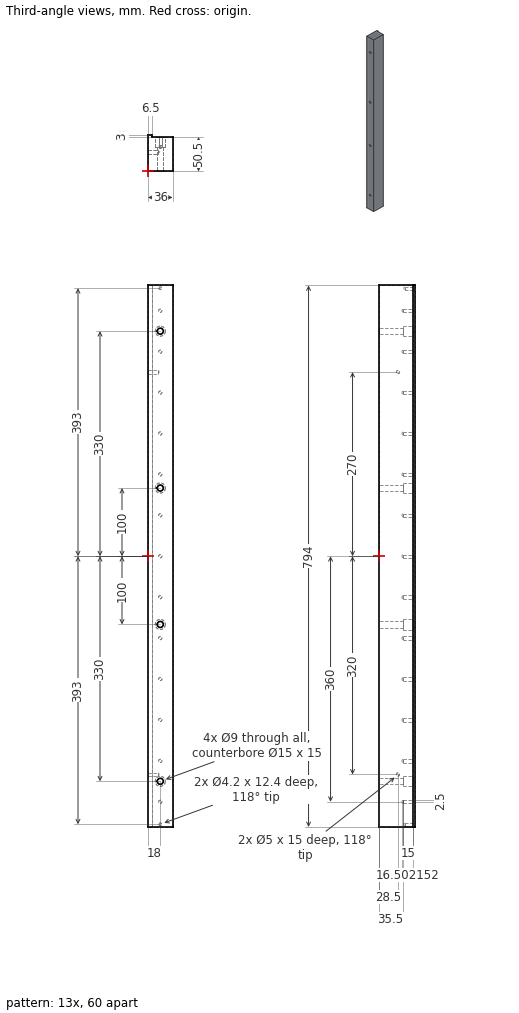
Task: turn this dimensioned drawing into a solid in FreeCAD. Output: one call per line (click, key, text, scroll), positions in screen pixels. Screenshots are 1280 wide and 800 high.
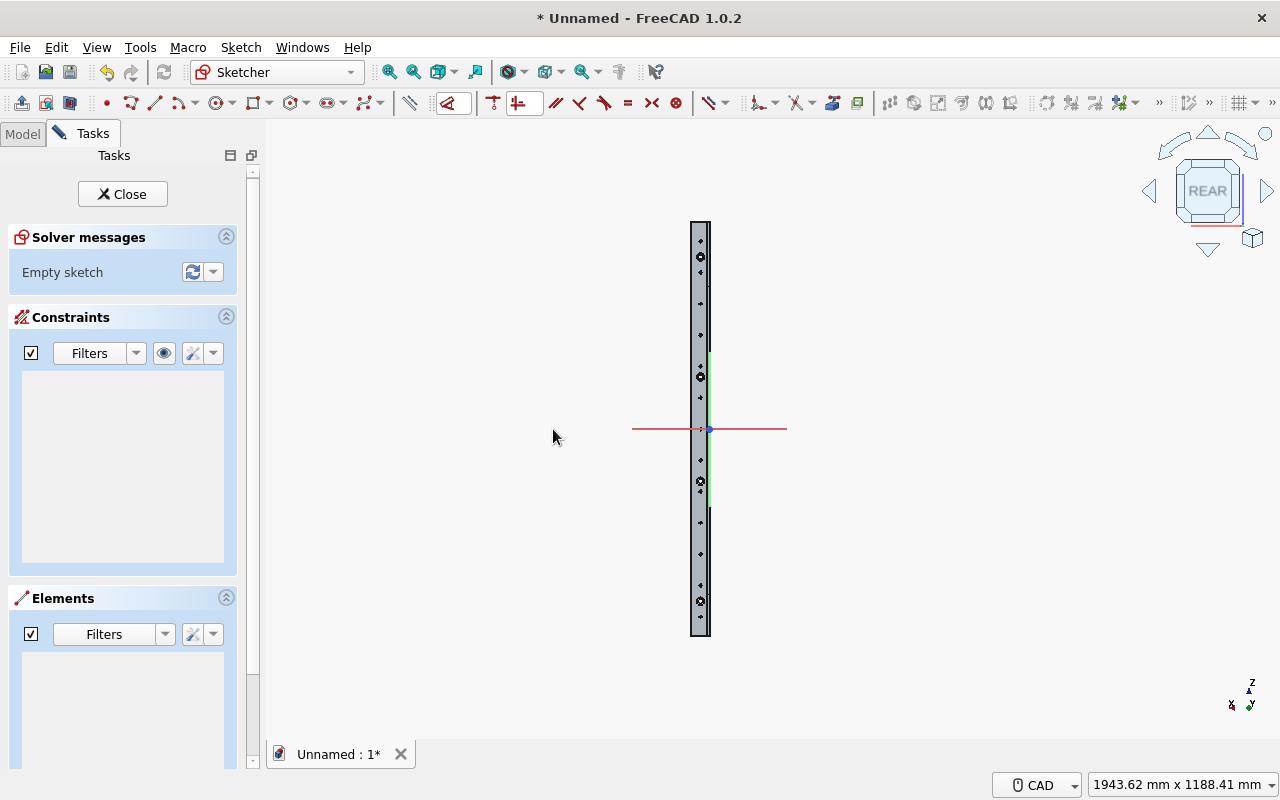
click(216, 104)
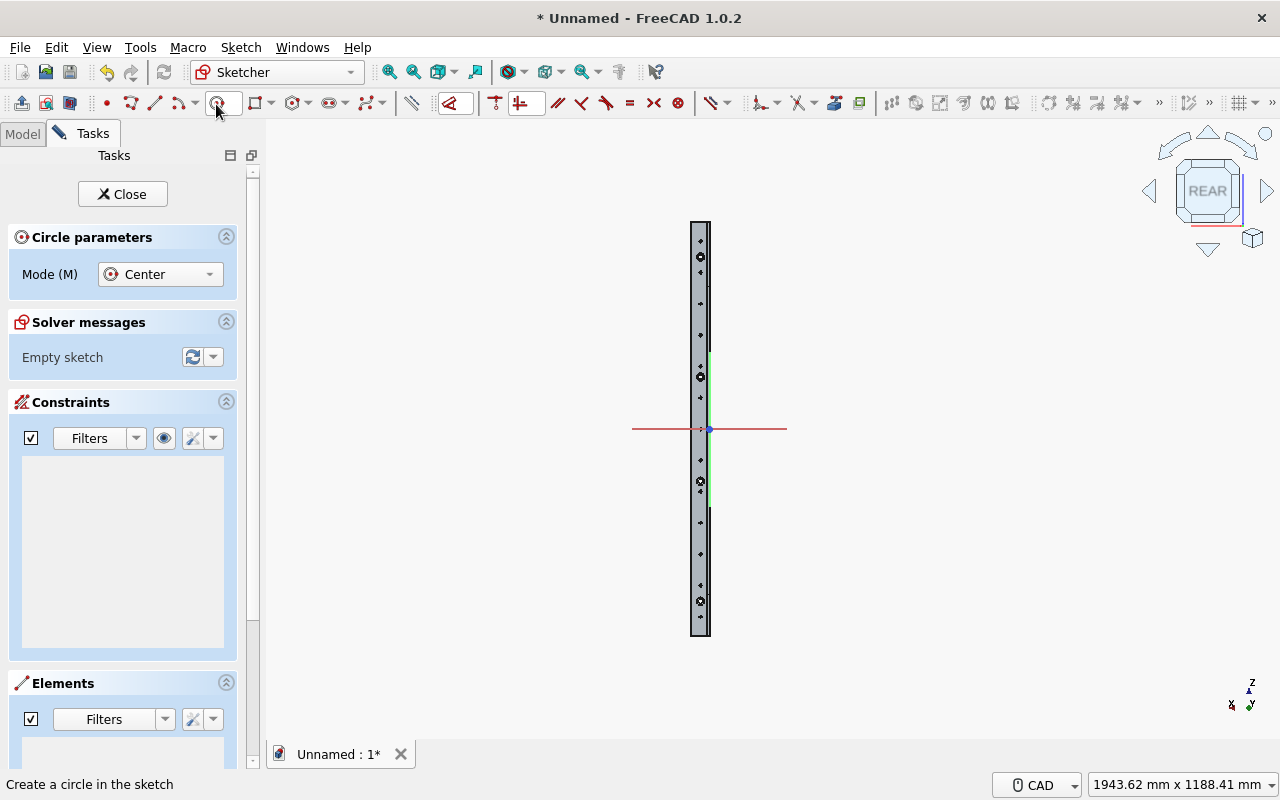
scroll(701, 634, up, 16)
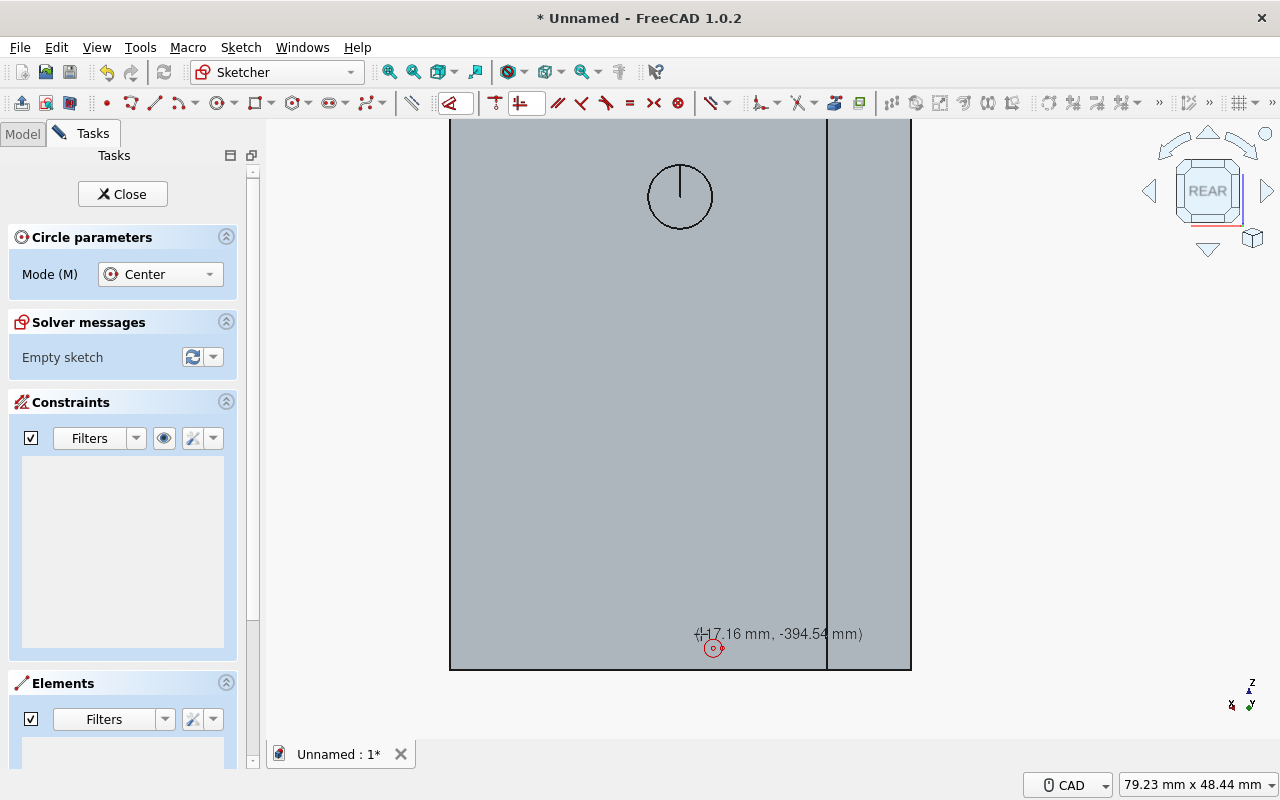
scroll(700, 683, down, 15)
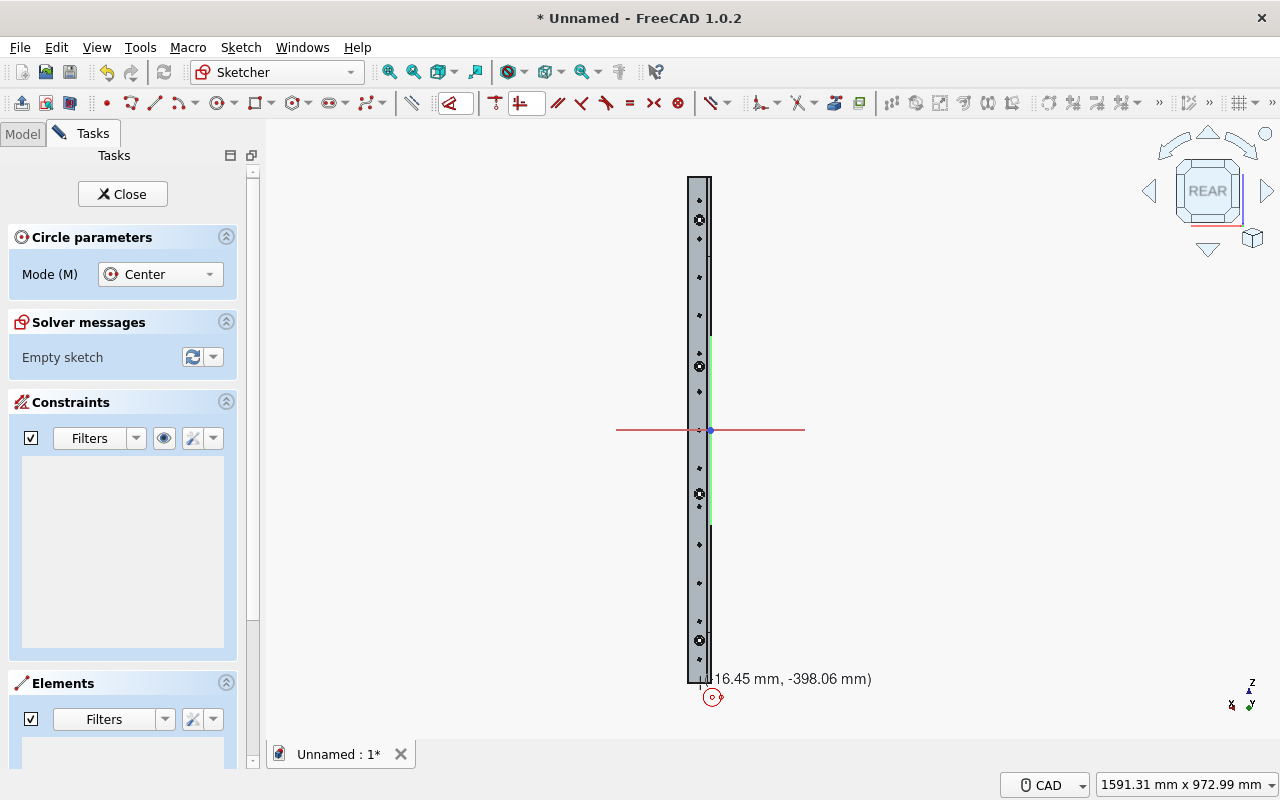
scroll(699, 681, up, 2)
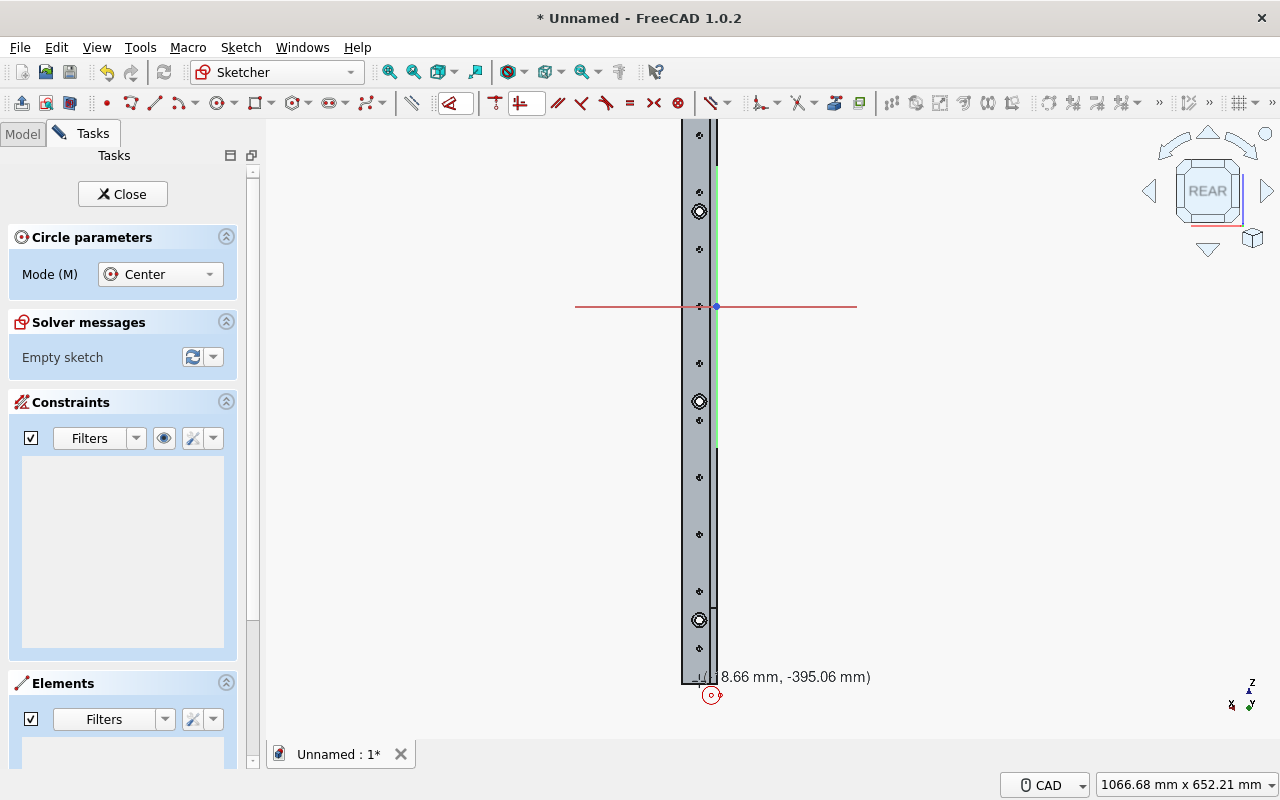
click(699, 680)
move(701, 679)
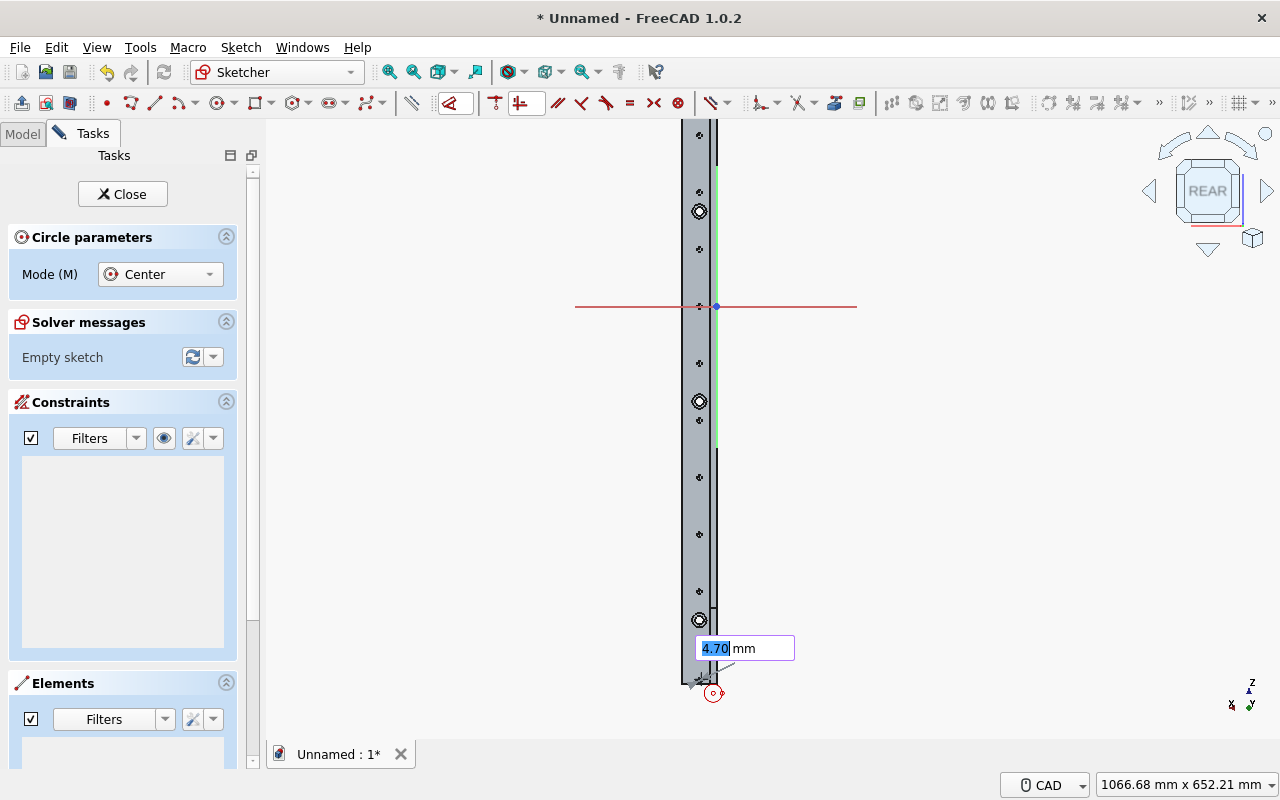
text(4.2)
key(Return)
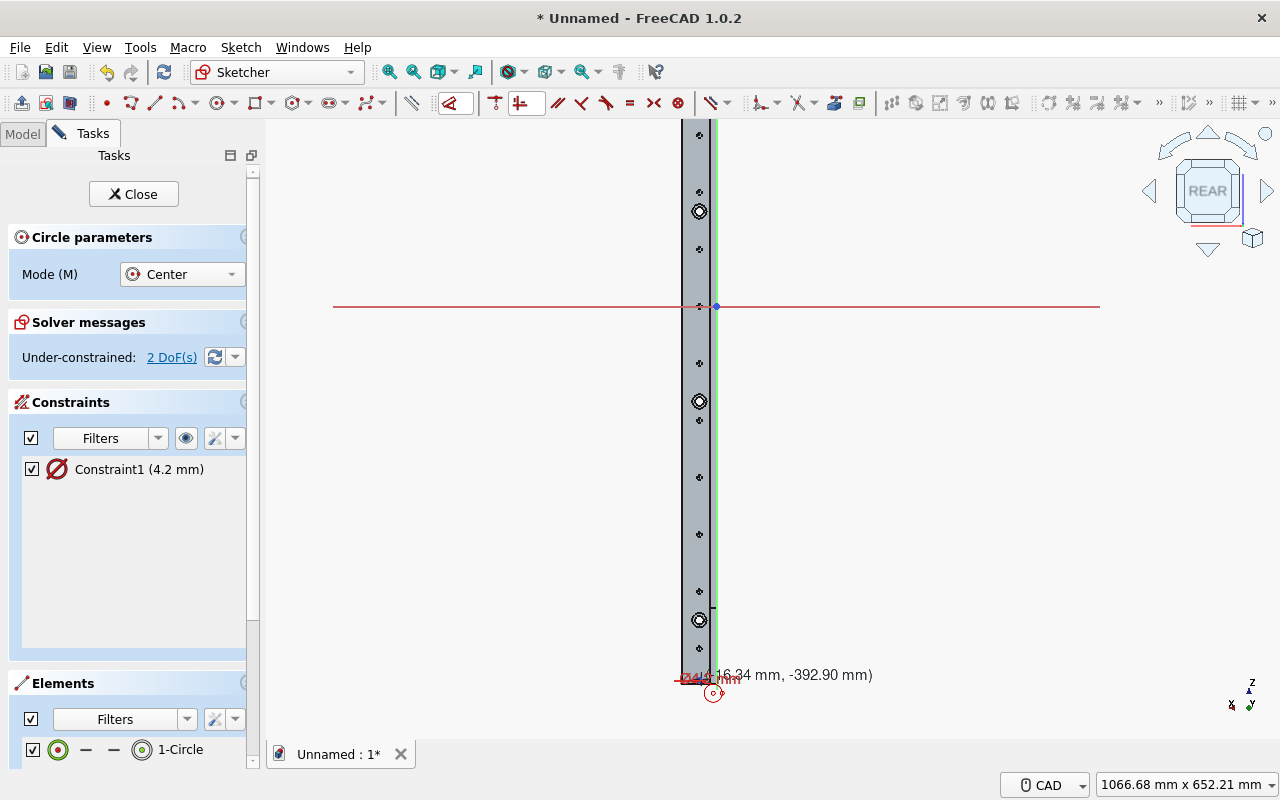
scroll(701, 578, down, 3)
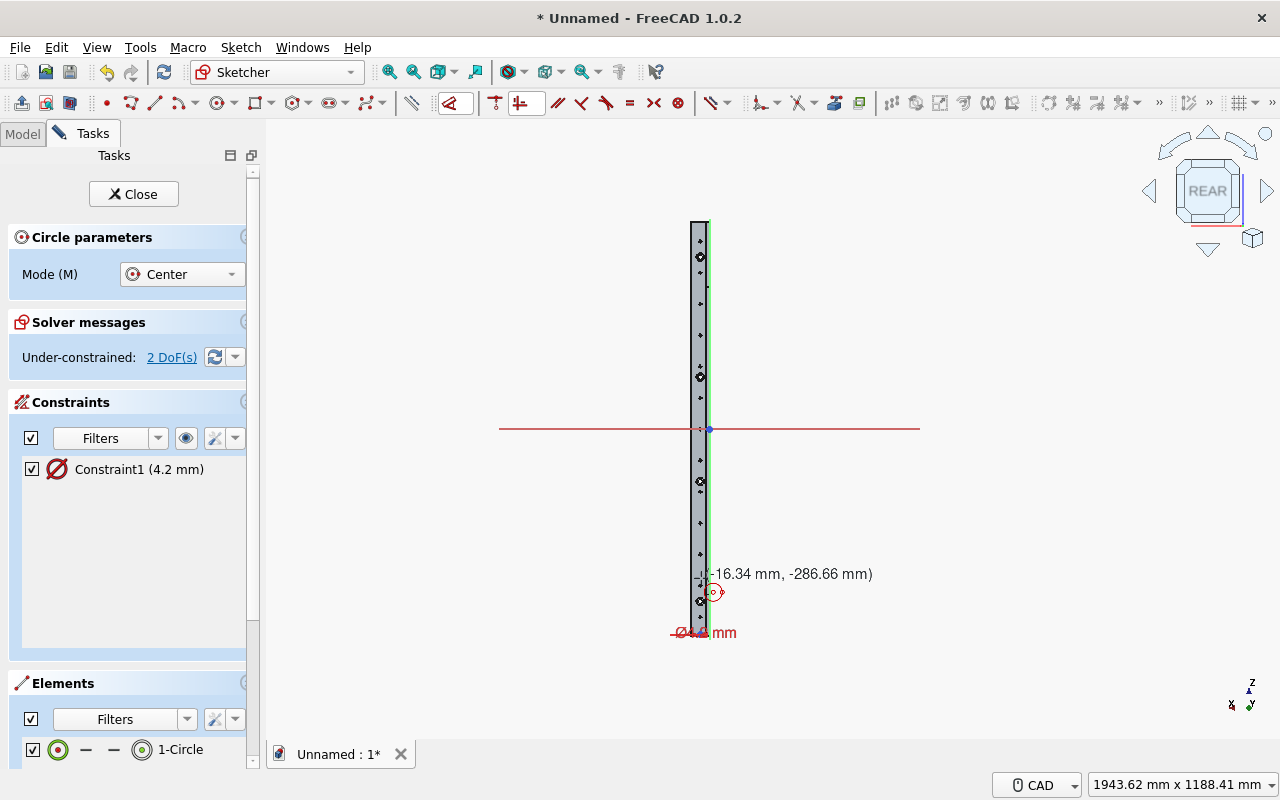
scroll(700, 224, up, 16)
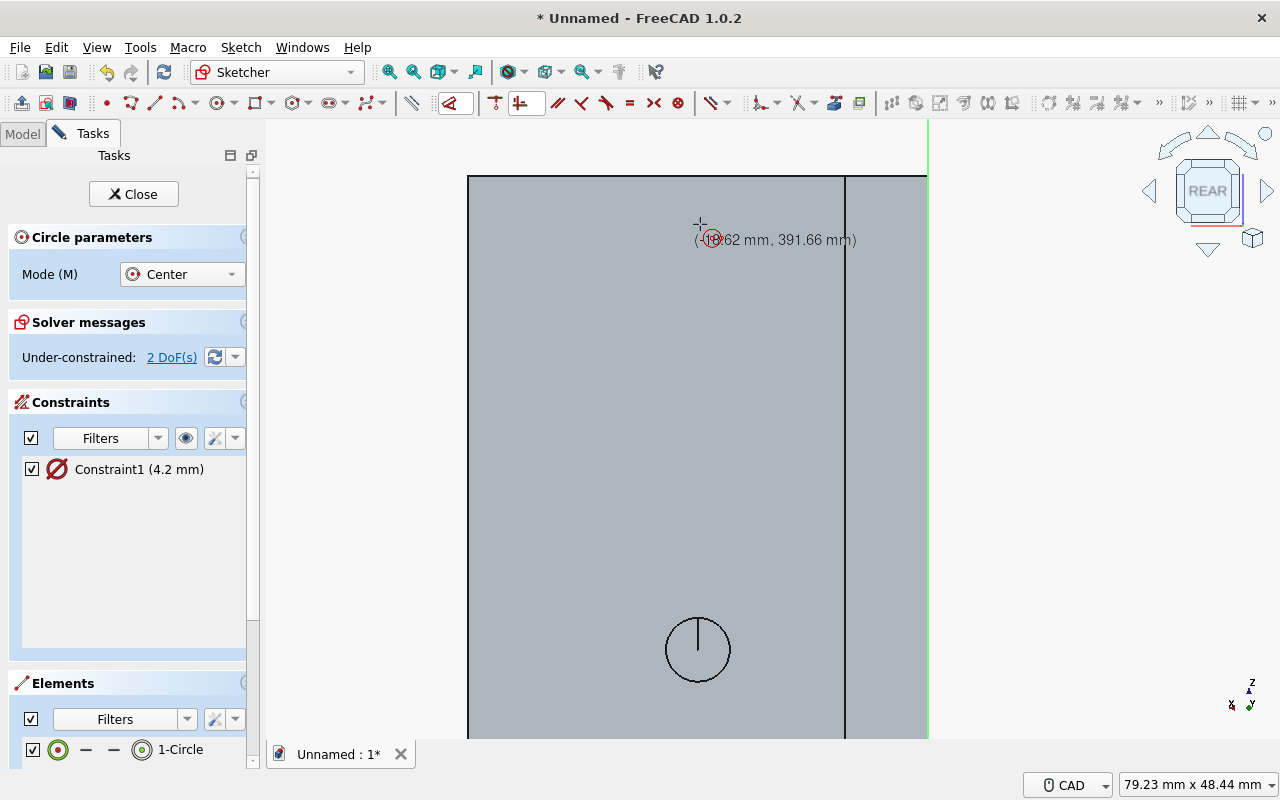
scroll(700, 176, down, 15)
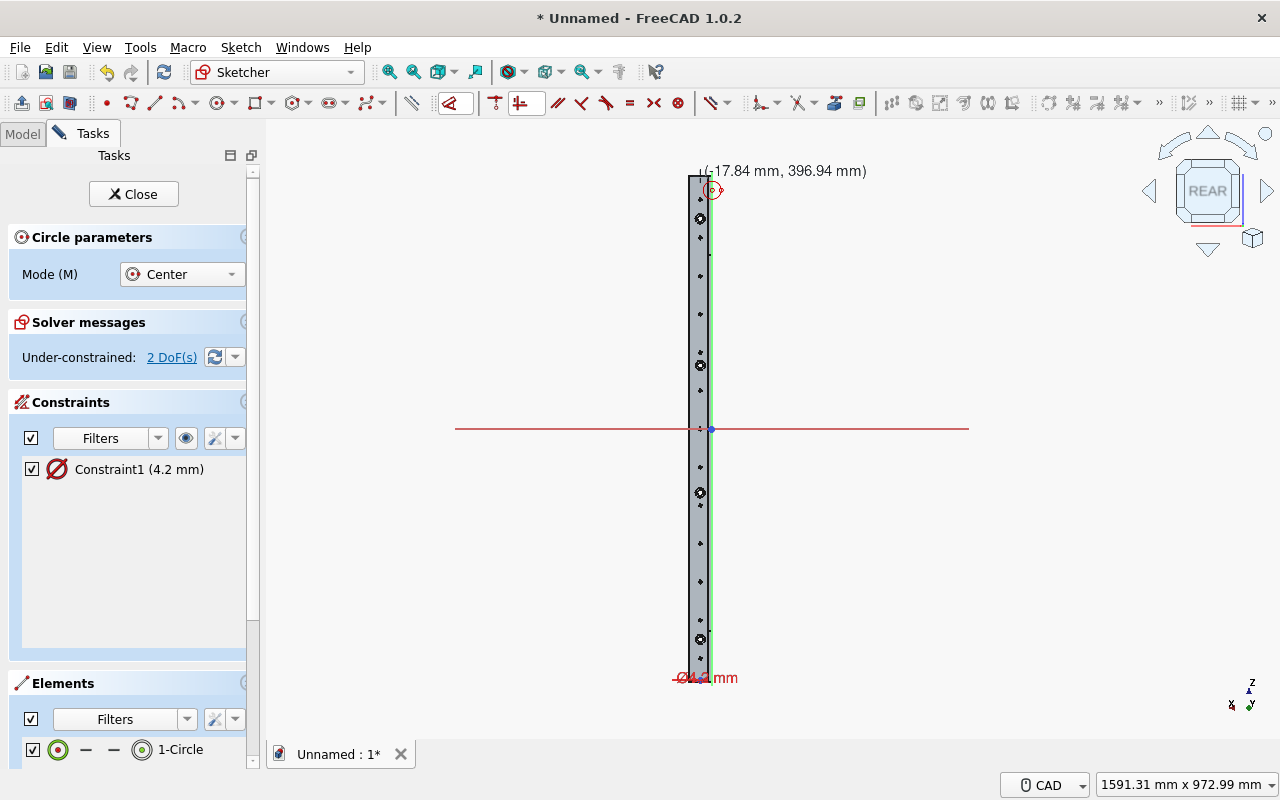
scroll(700, 179, up, 2)